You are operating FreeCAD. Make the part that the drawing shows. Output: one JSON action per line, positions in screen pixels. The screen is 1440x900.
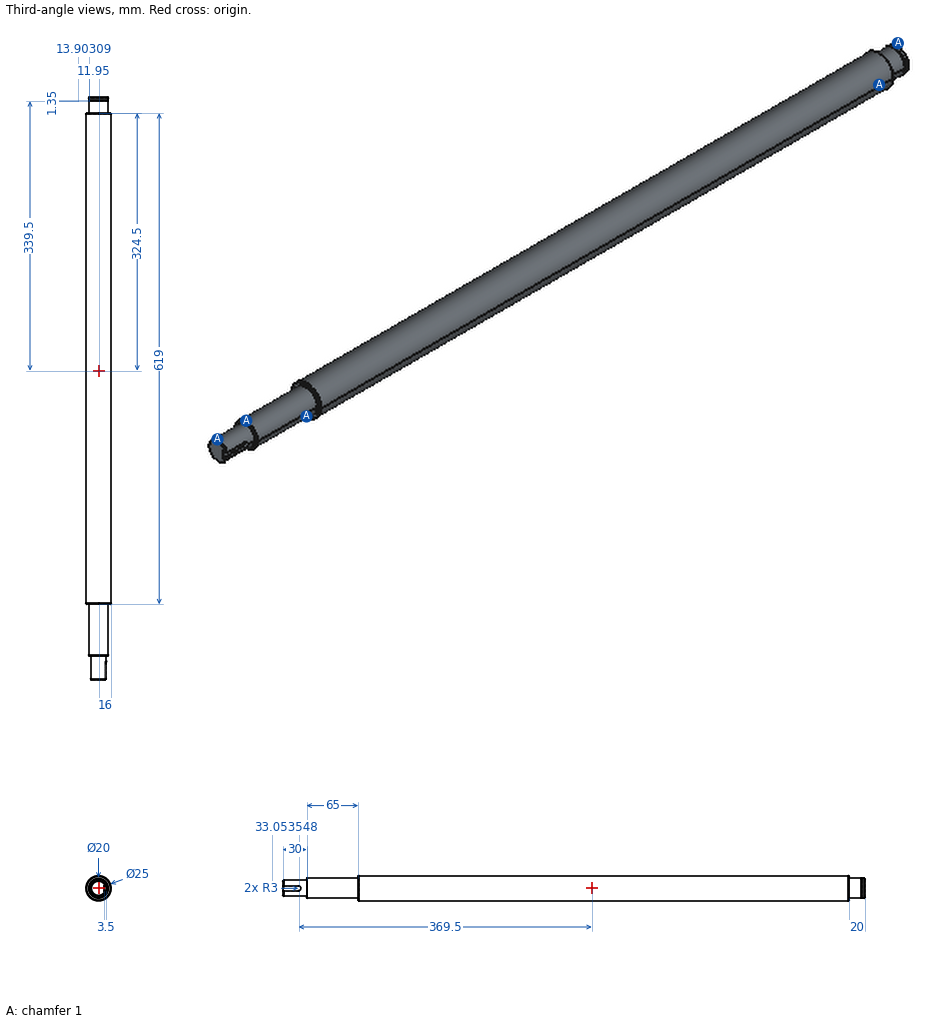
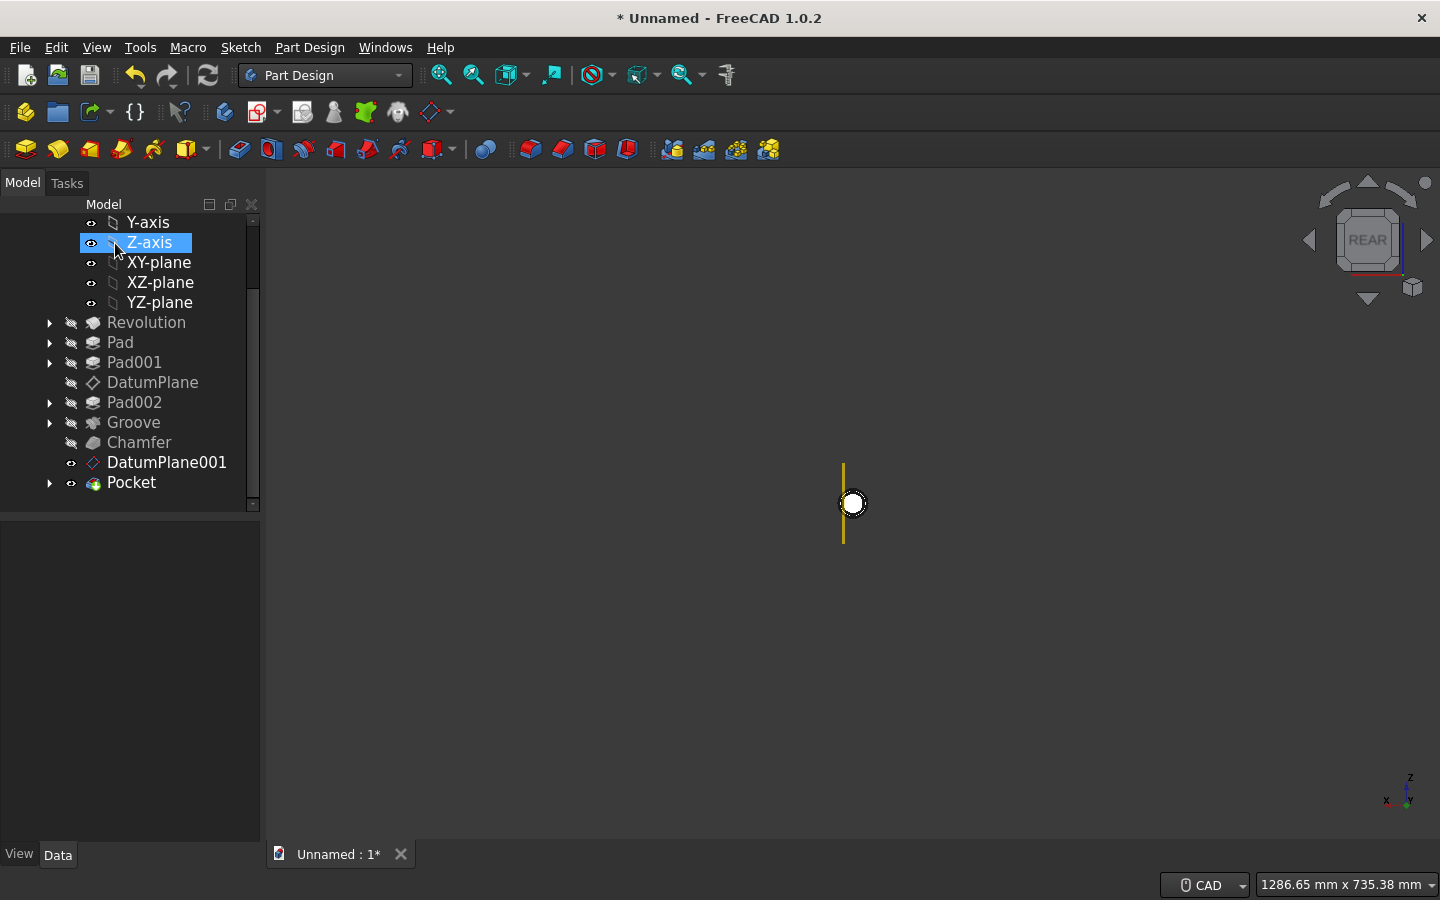
{"action": "left_click", "coordinate": [116, 463]}
{"action": "key", "text": "space"}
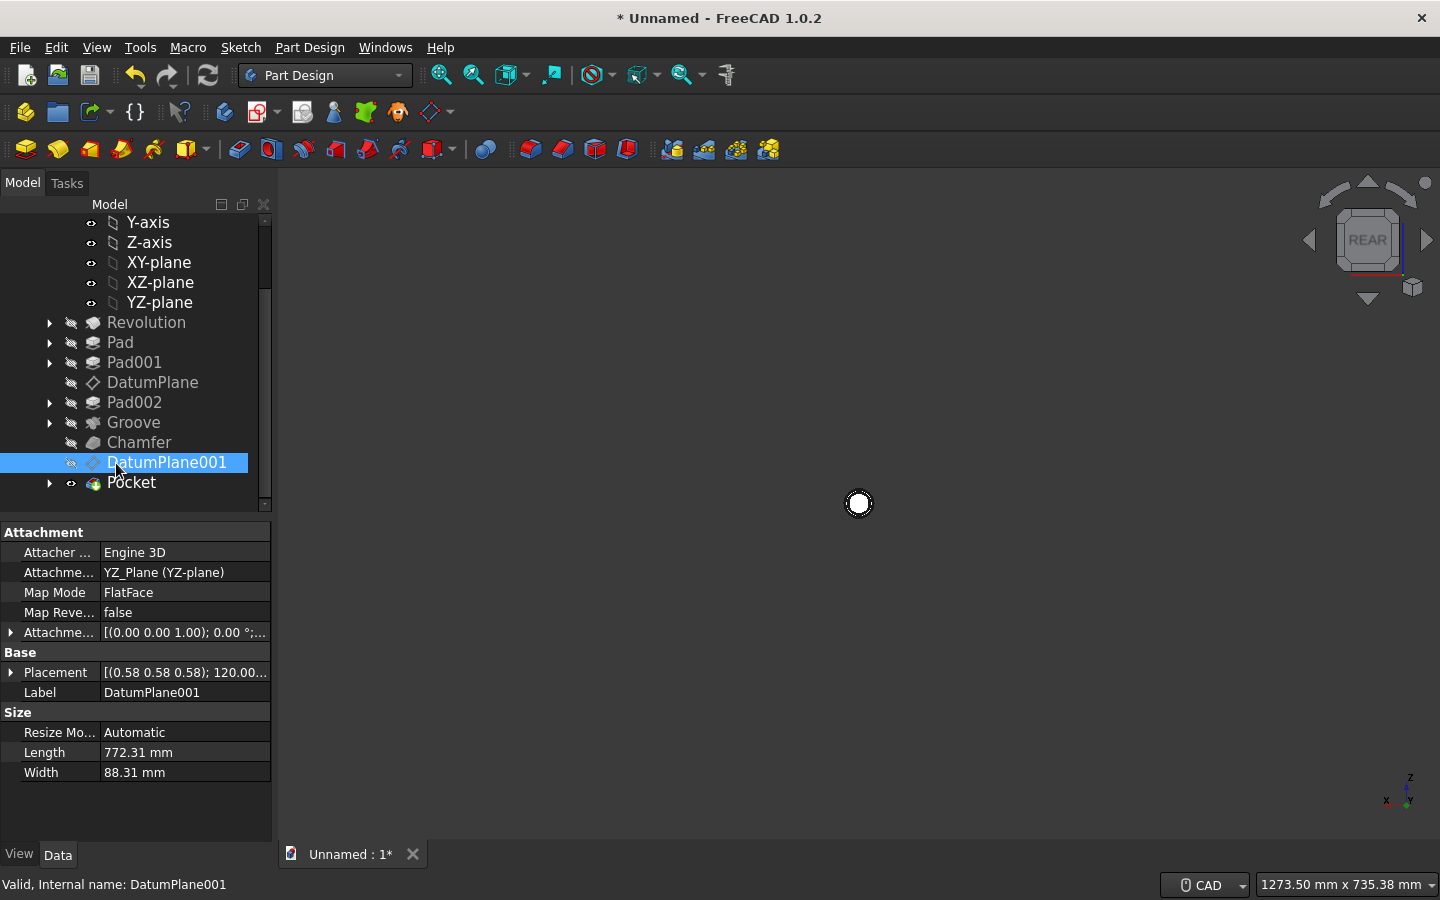
{"action": "key", "text": "0"}